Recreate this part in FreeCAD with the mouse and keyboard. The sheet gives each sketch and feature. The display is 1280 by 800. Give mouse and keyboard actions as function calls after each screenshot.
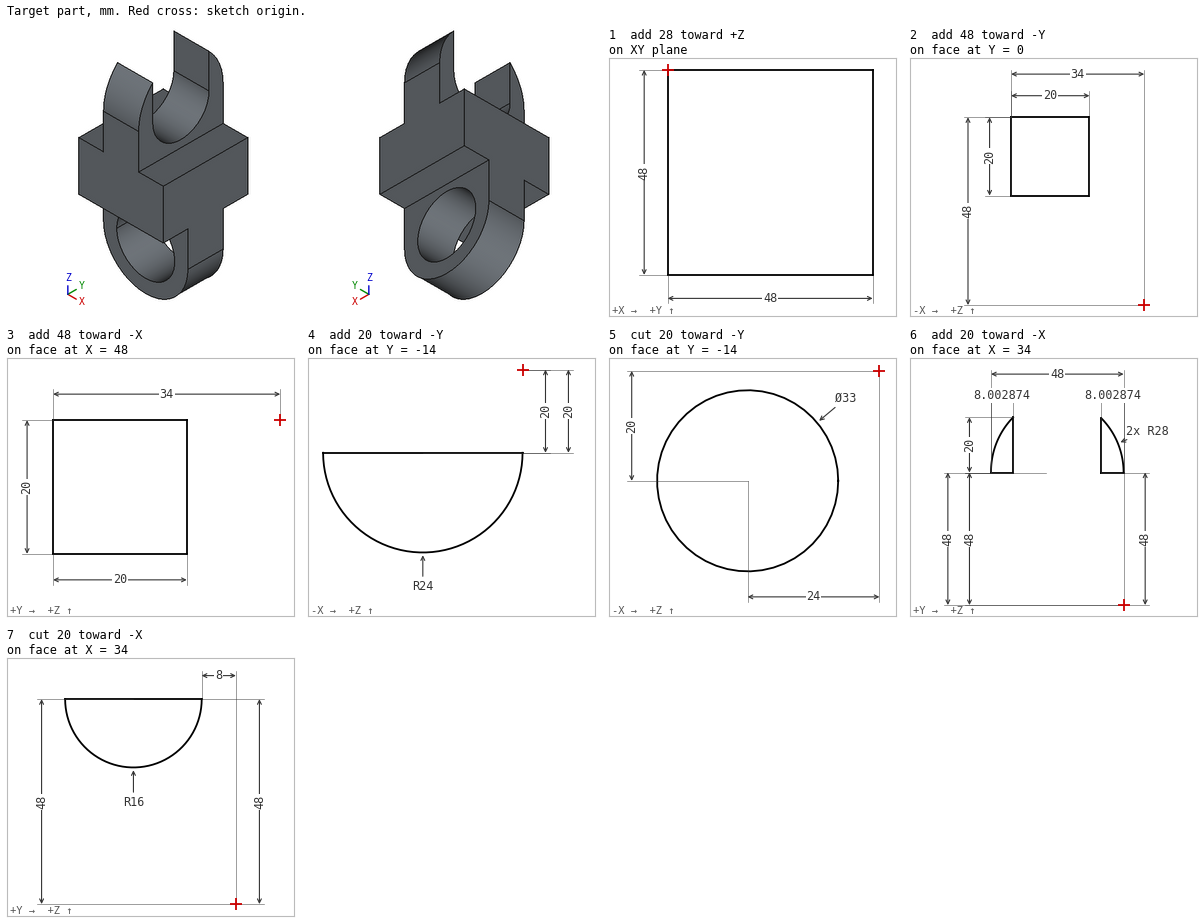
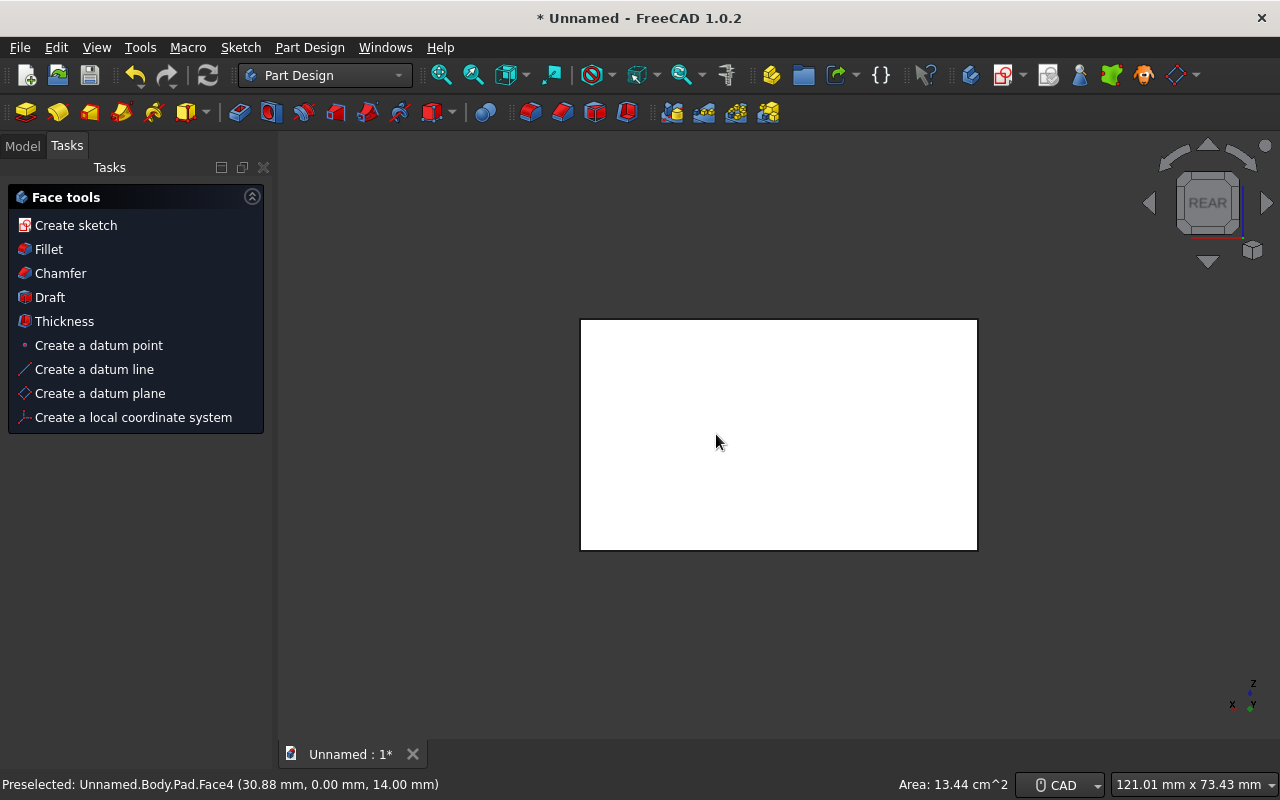
click(1004, 76)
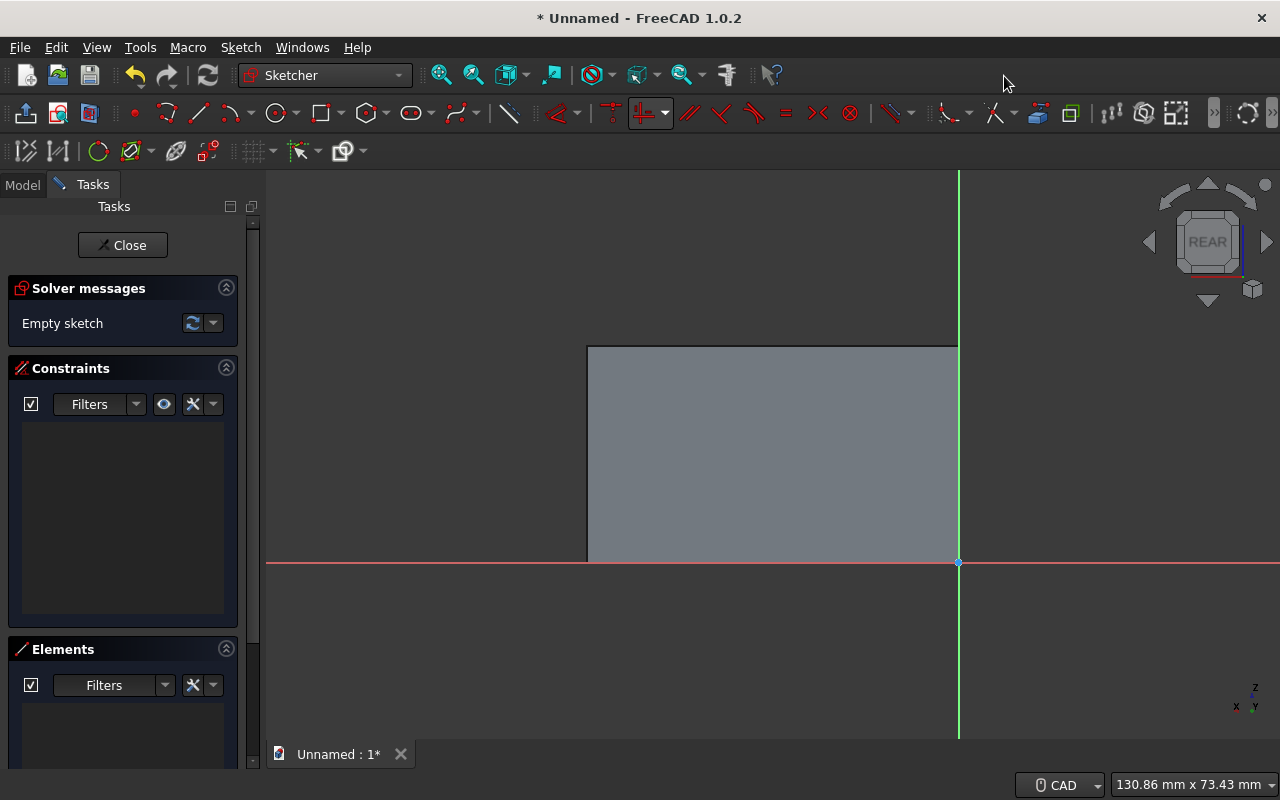
scroll(294, 711, down, 1)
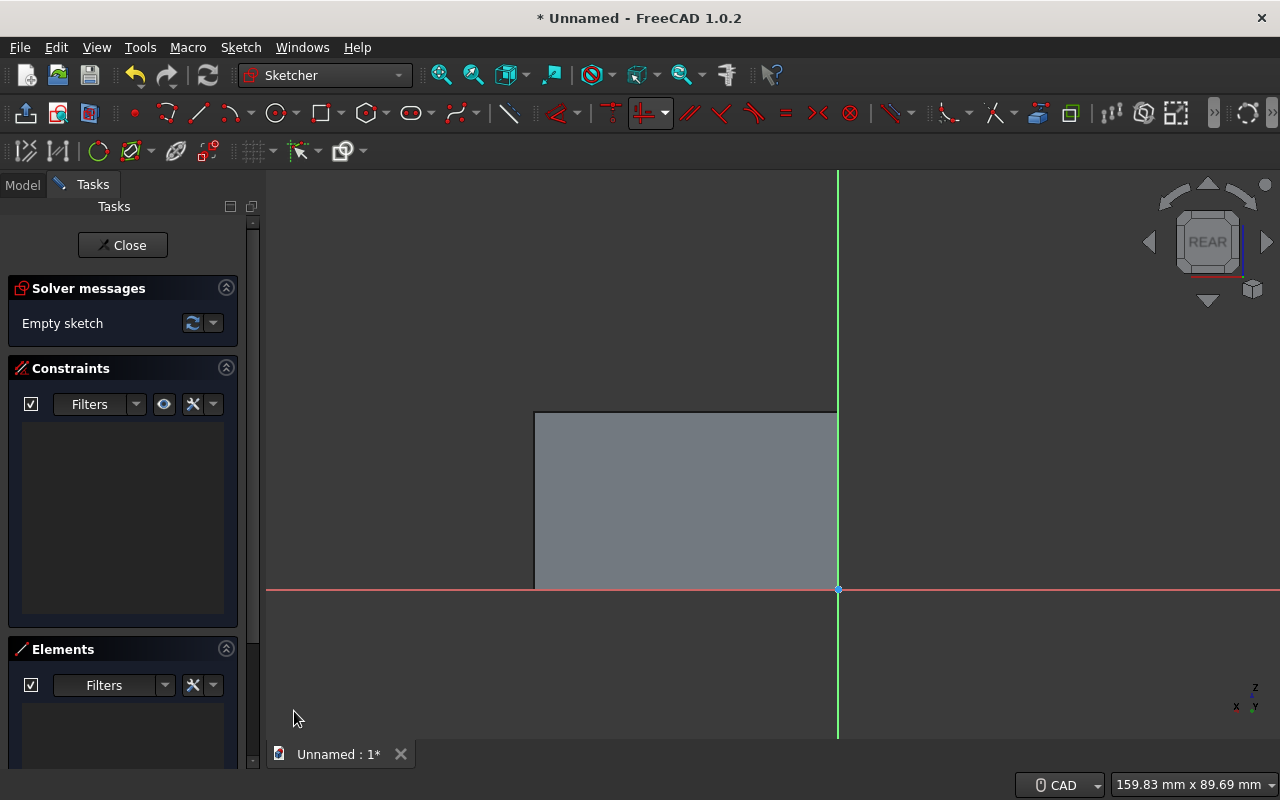
click(322, 114)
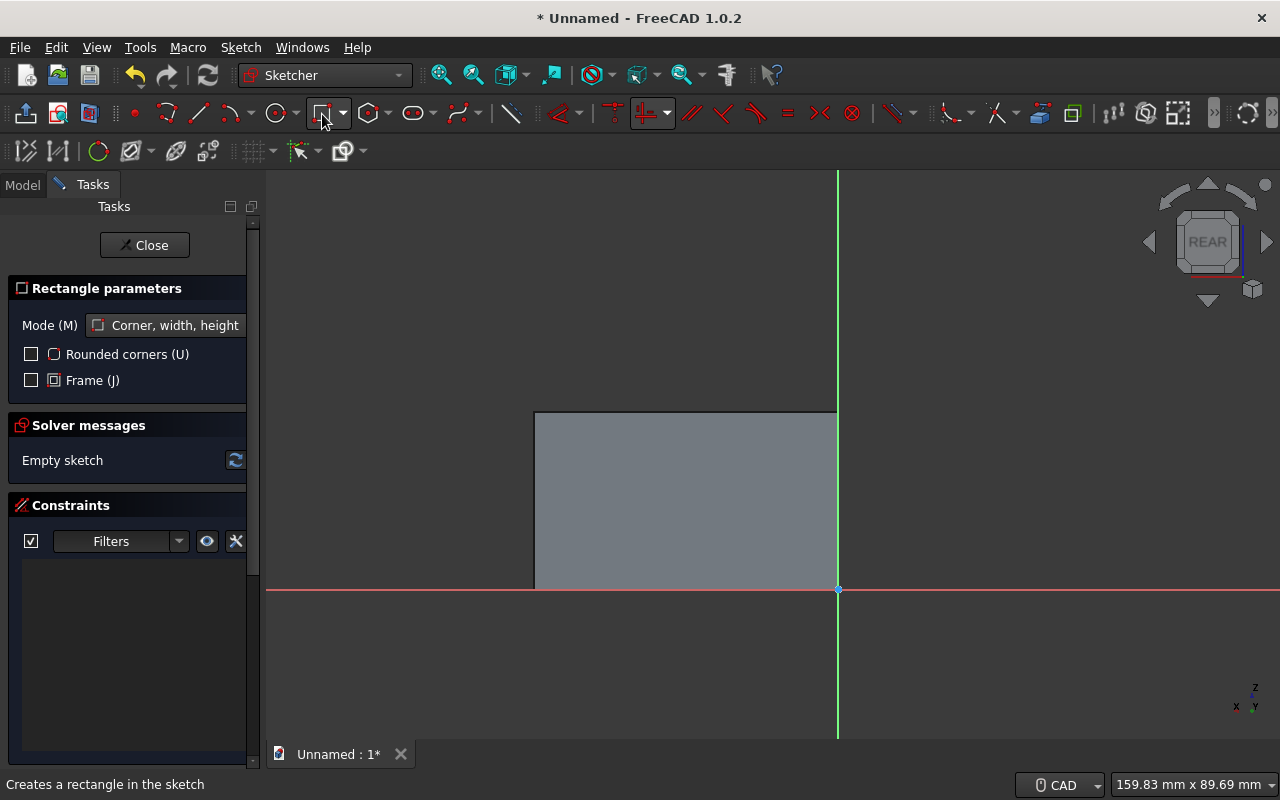
click(623, 285)
click(750, 412)
key(Escape)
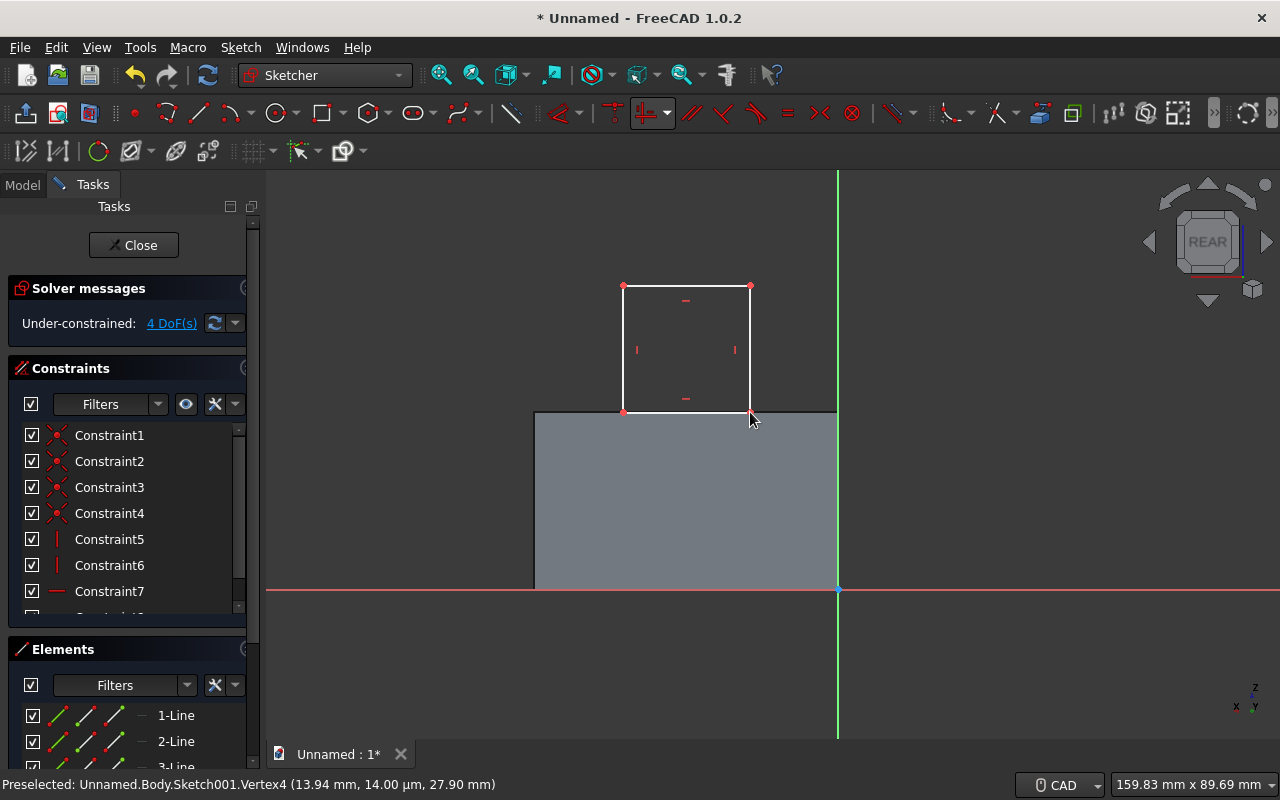
click(558, 114)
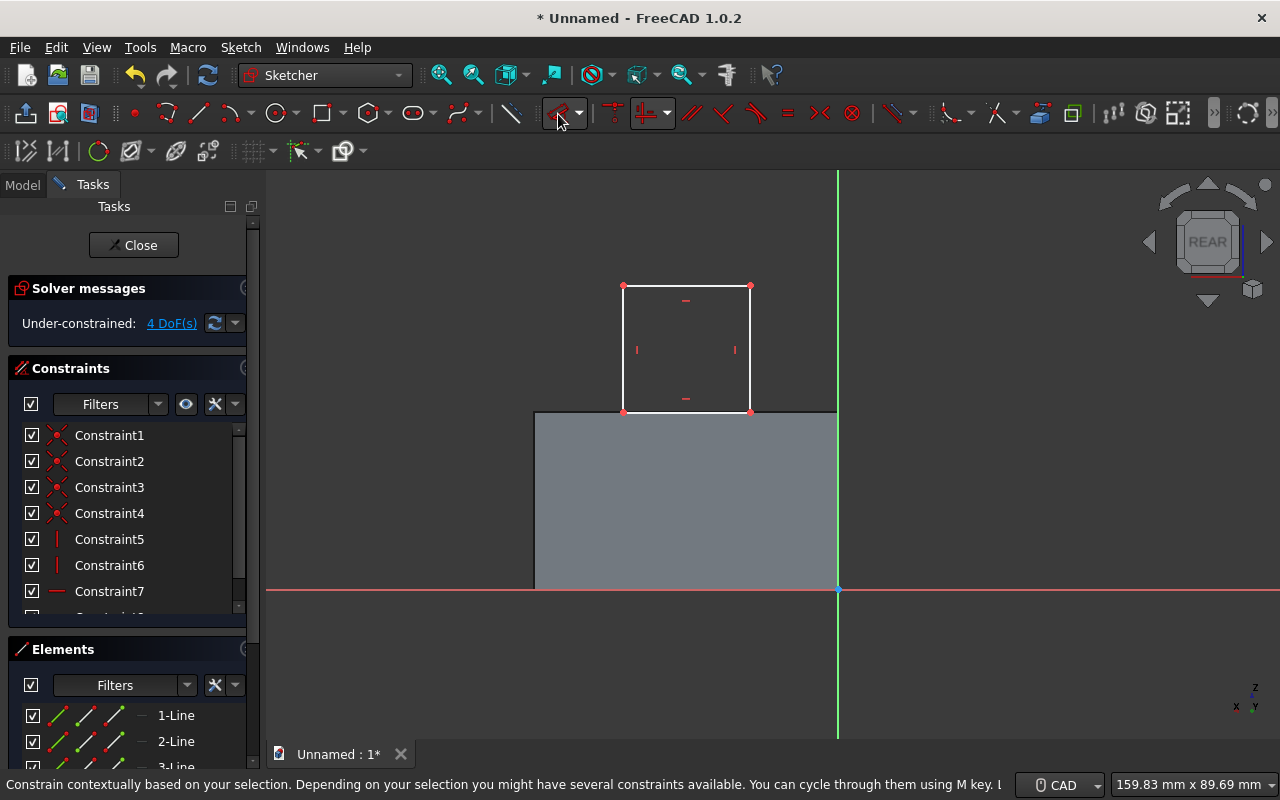
click(623, 324)
click(589, 349)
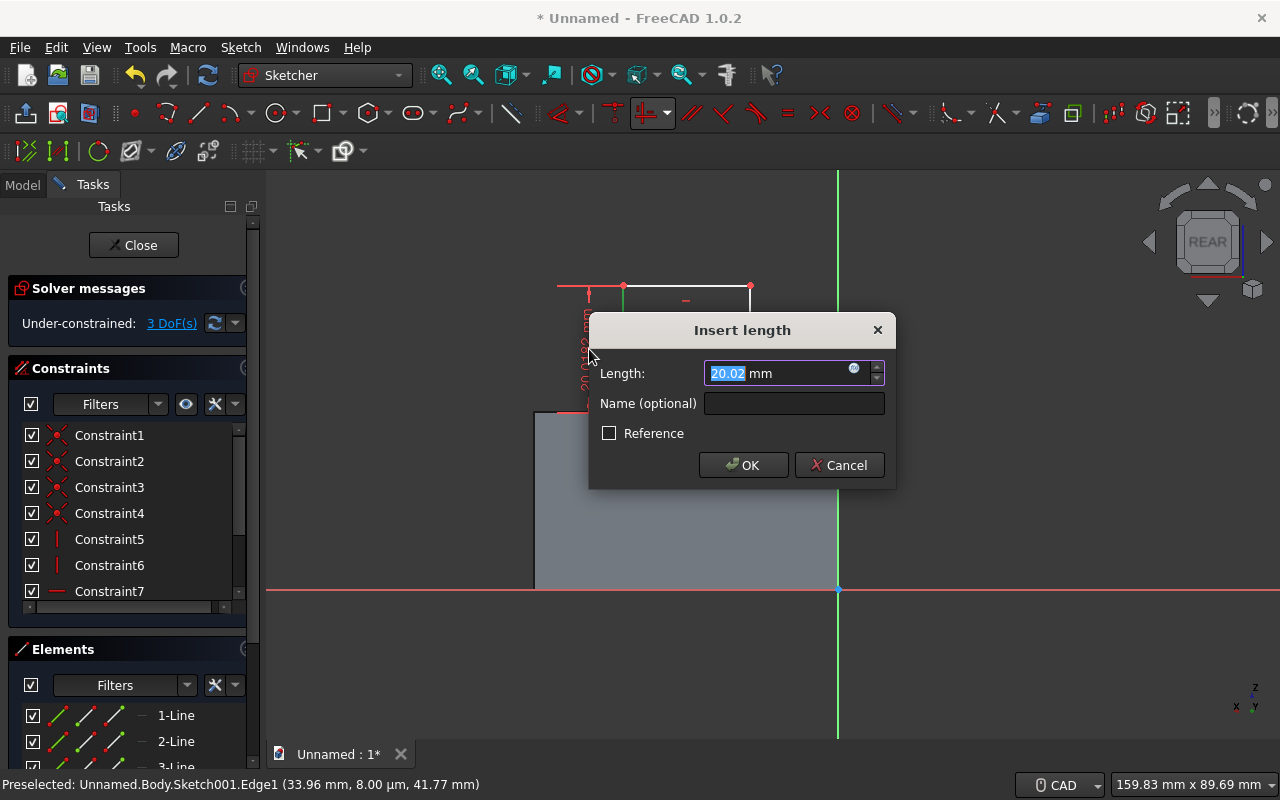
text(20)
key(Return)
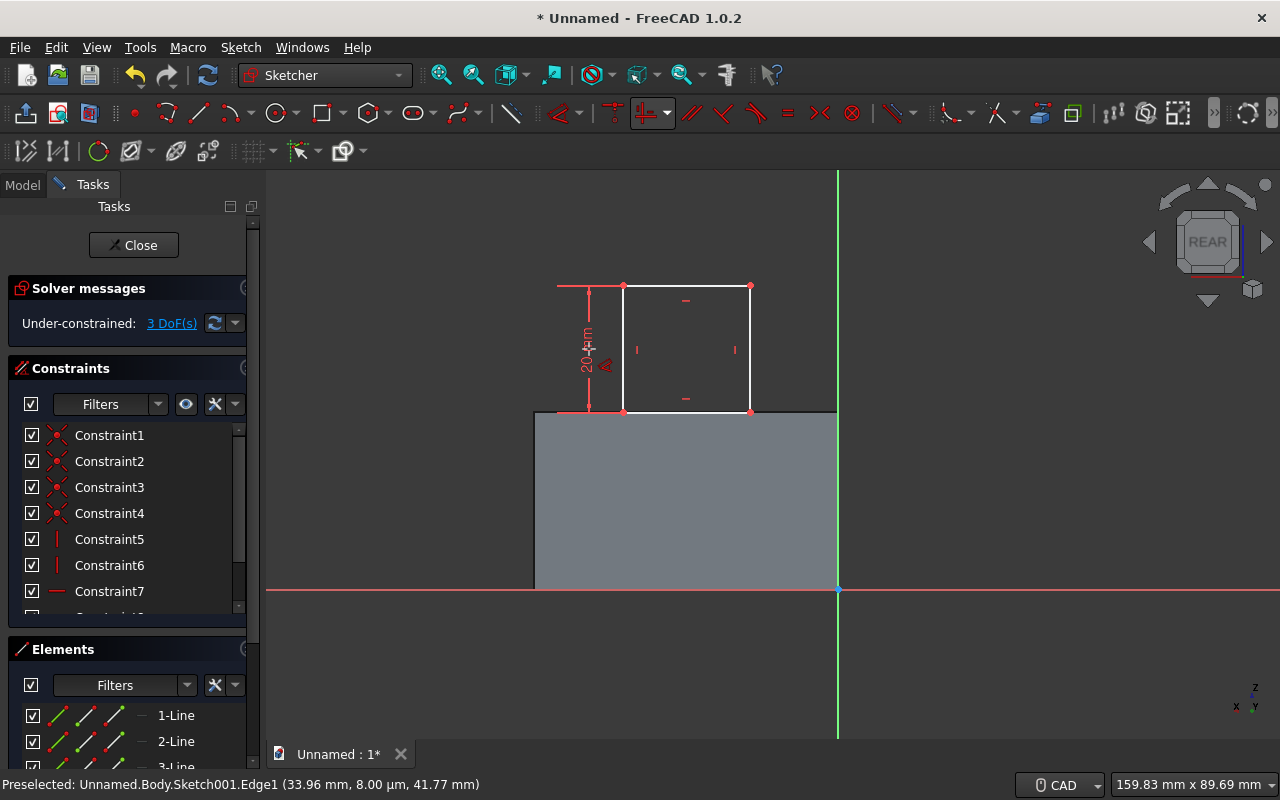
click(661, 413)
click(686, 379)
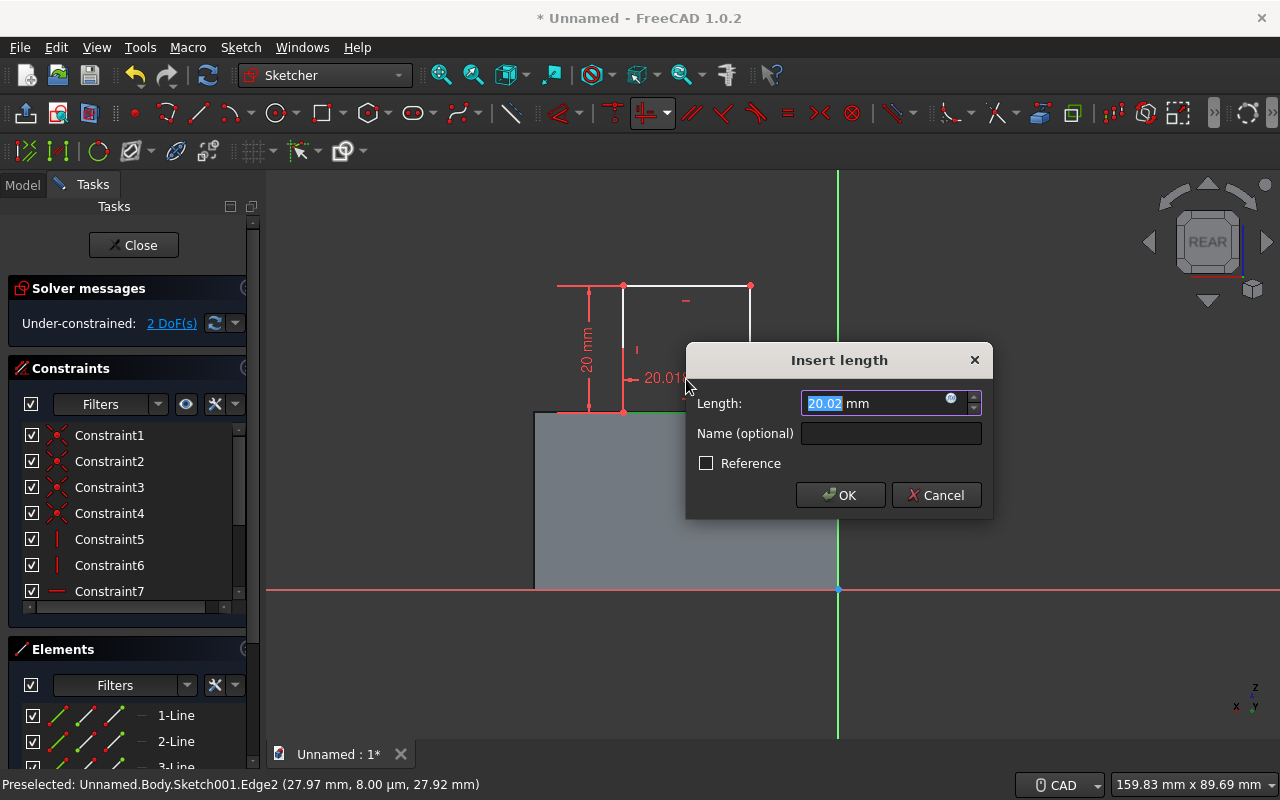
text(20)
key(Return)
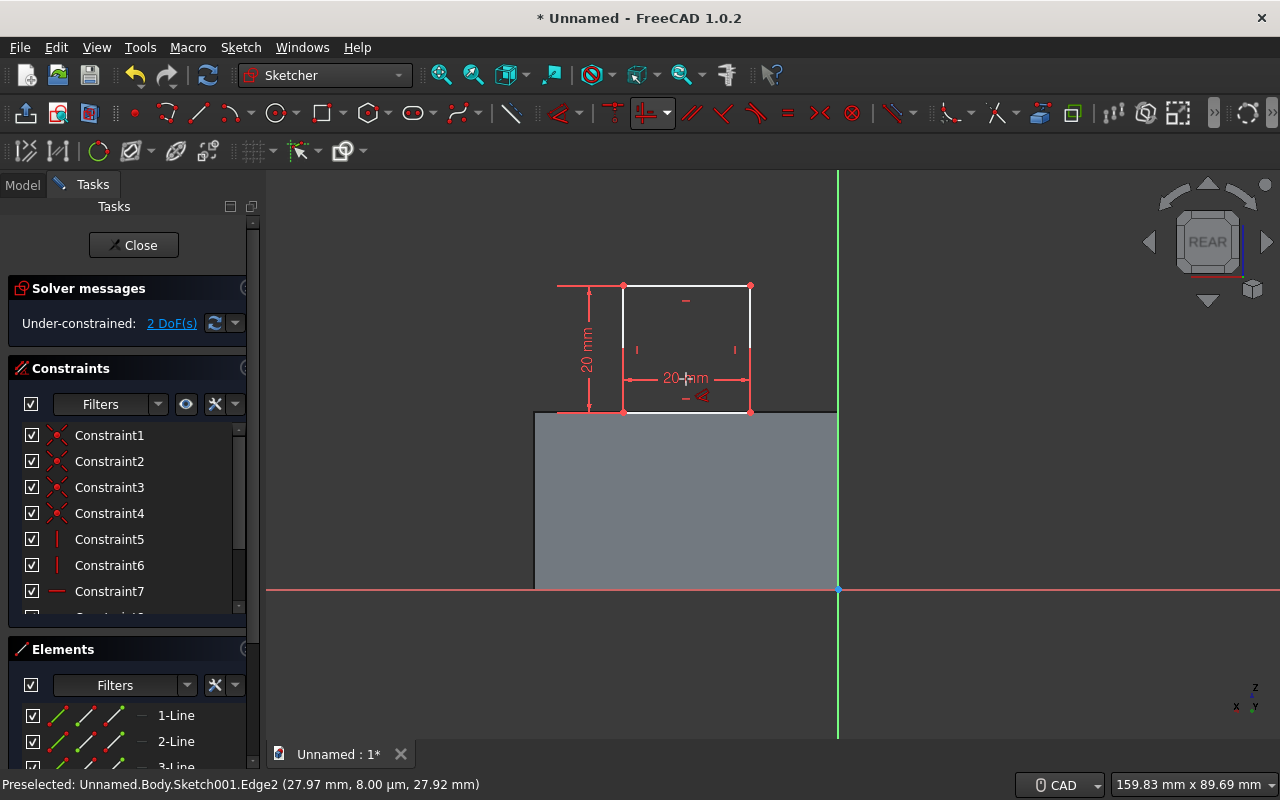
click(623, 286)
click(731, 624)